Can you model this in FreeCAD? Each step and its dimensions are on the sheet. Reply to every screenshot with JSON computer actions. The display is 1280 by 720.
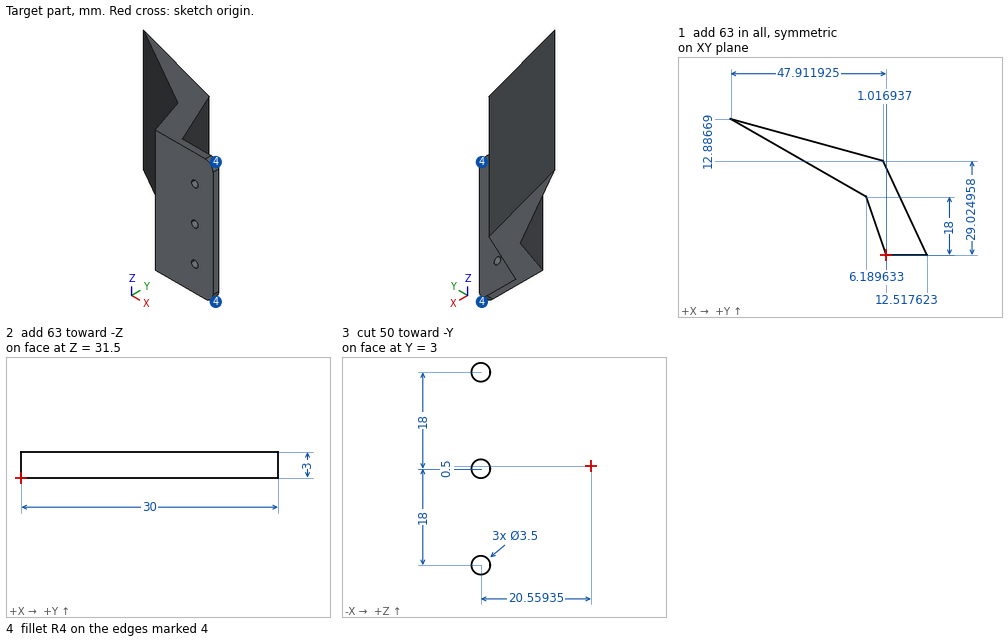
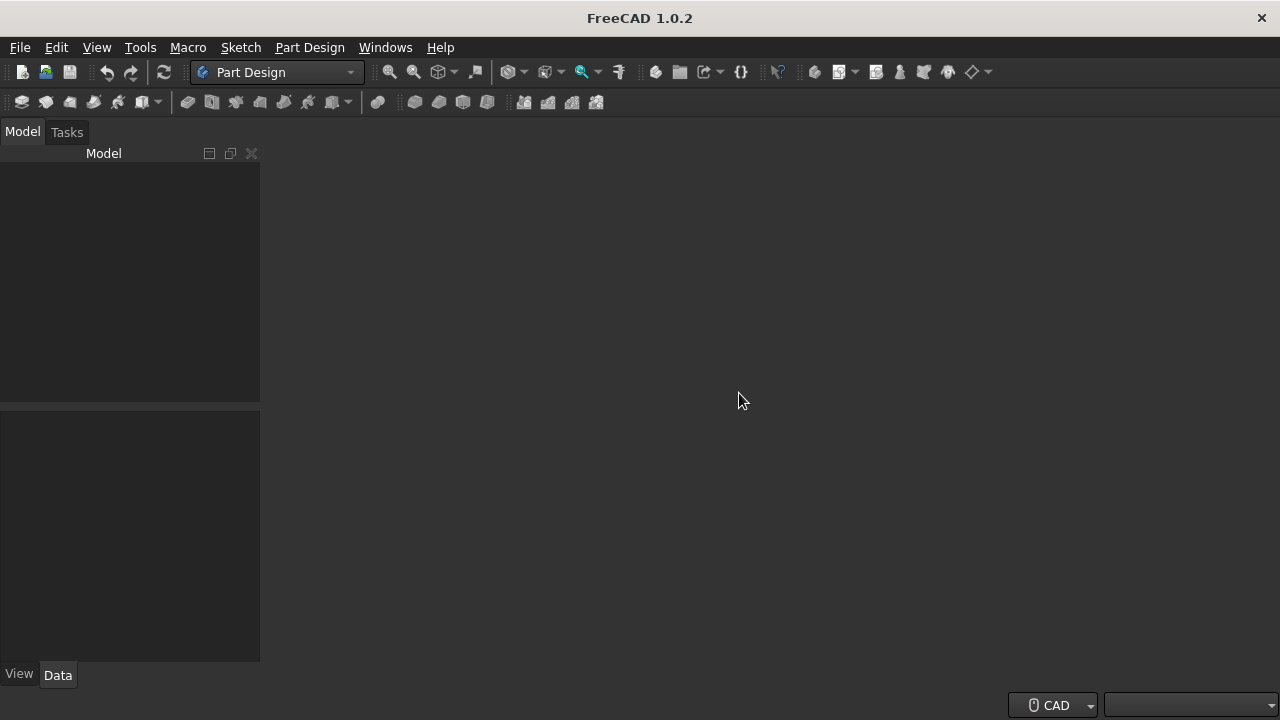
{"action": "key", "text": "ctrl+n"}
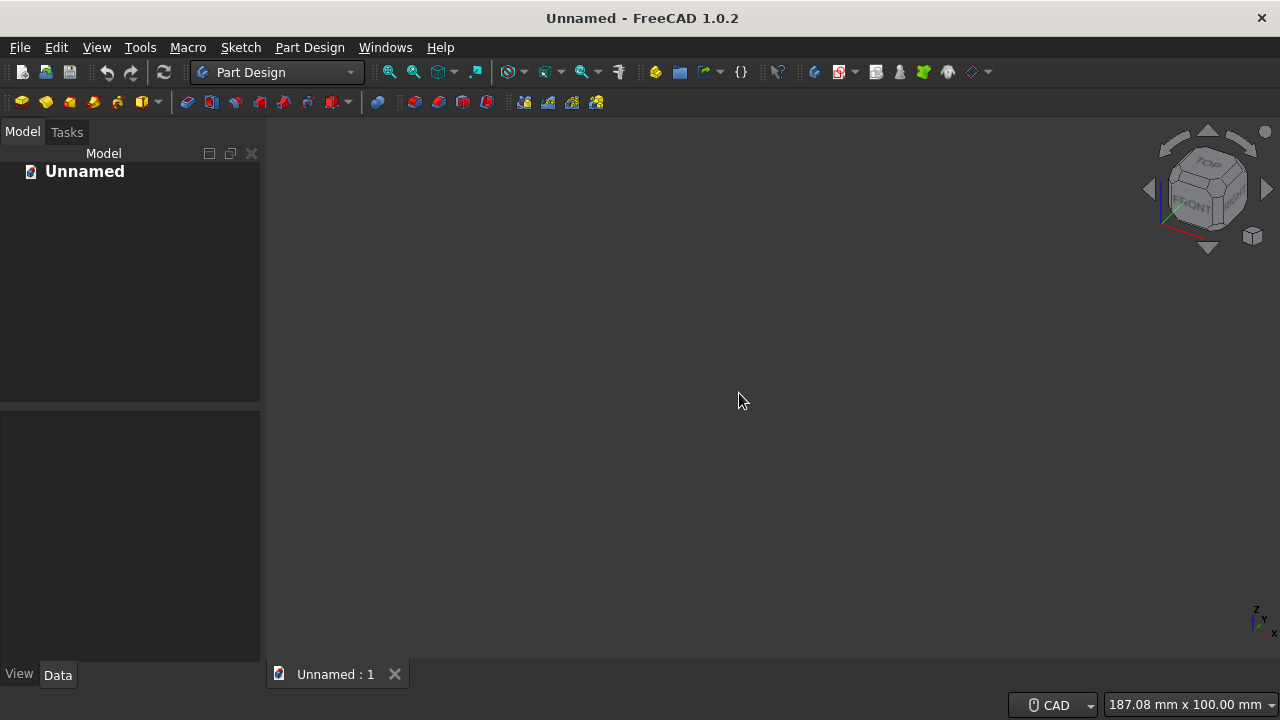
{"action": "left_click", "coordinate": [840, 72]}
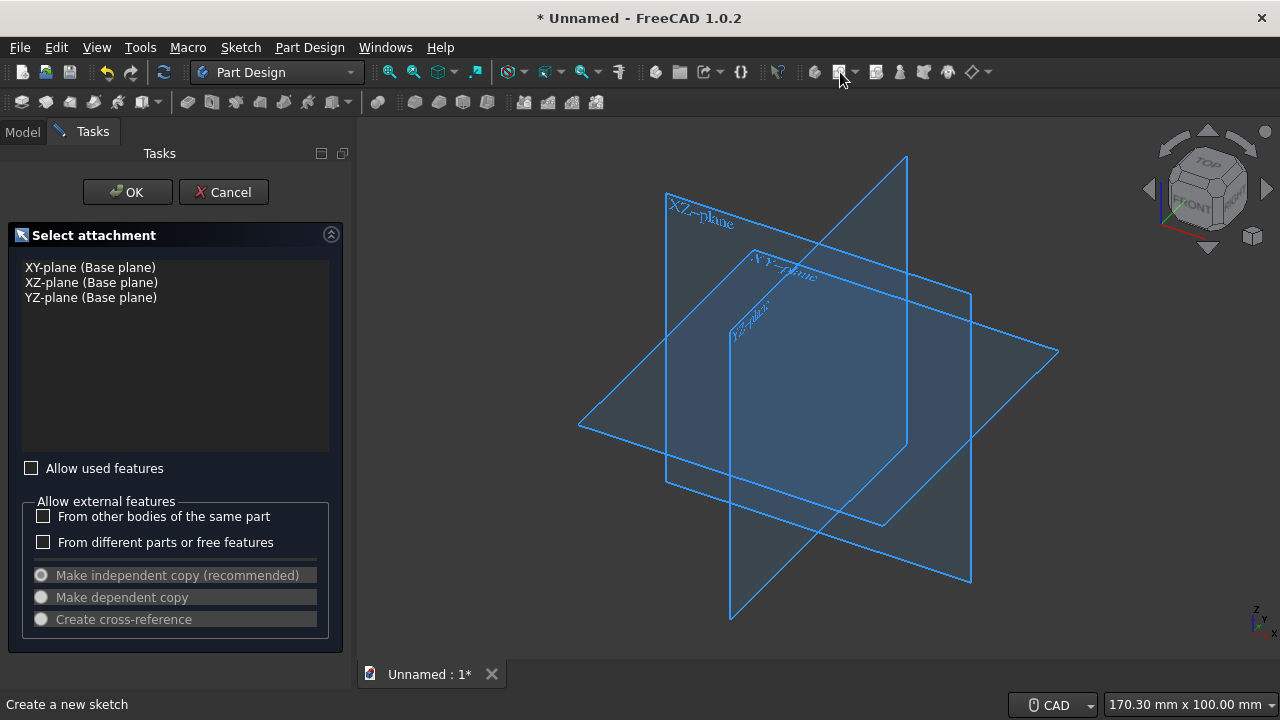
{"action": "left_click", "coordinate": [82, 268]}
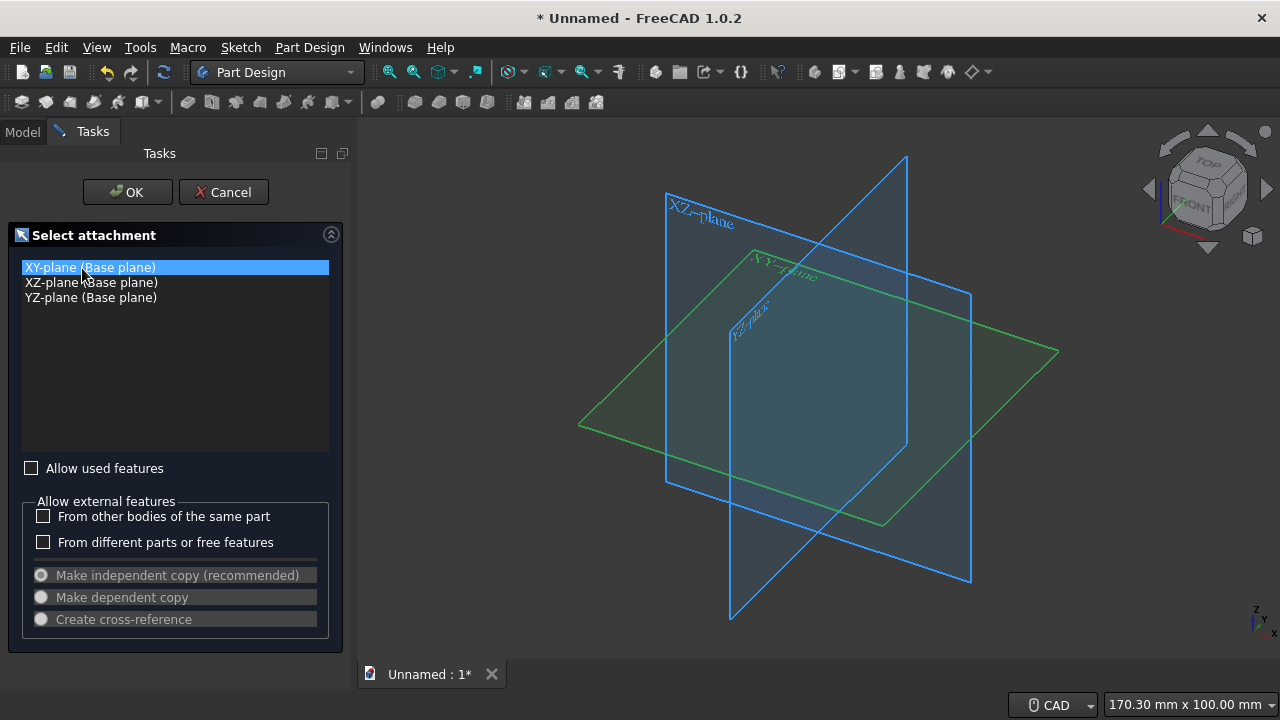
{"action": "left_click", "coordinate": [128, 192]}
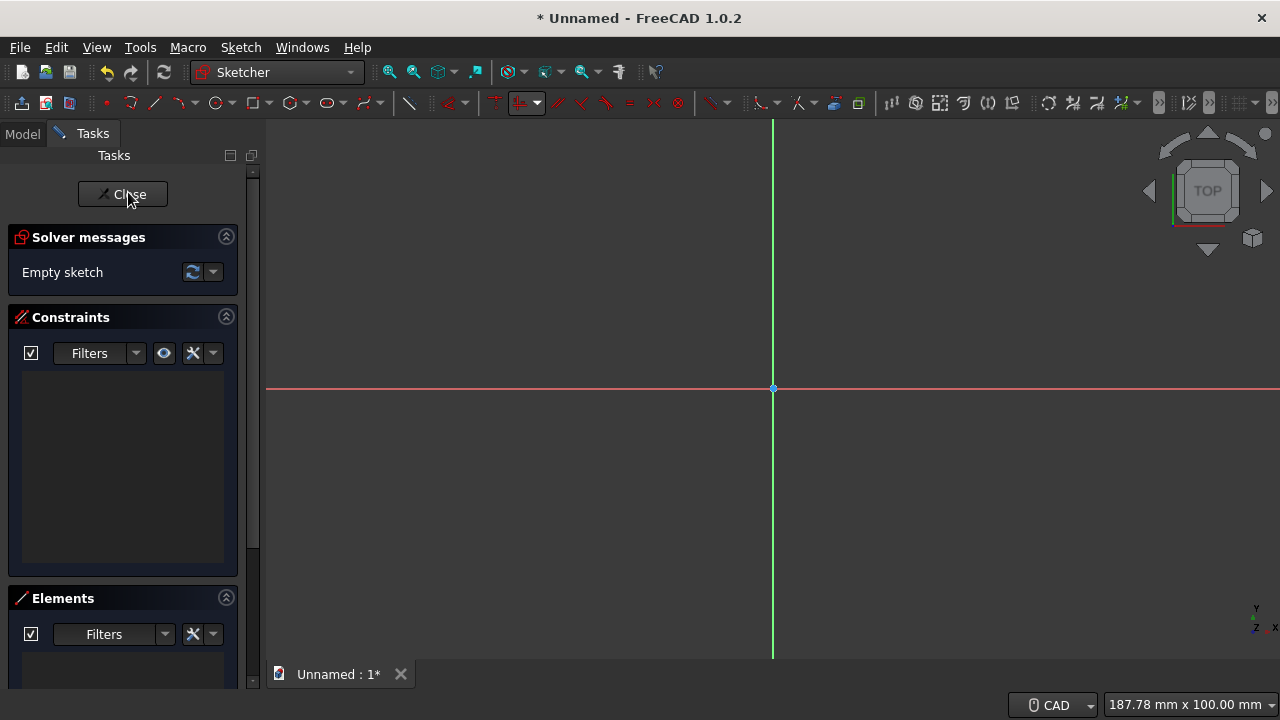
{"action": "scroll", "coordinate": [827, 631], "scroll_direction": "down", "scroll_amount": 1}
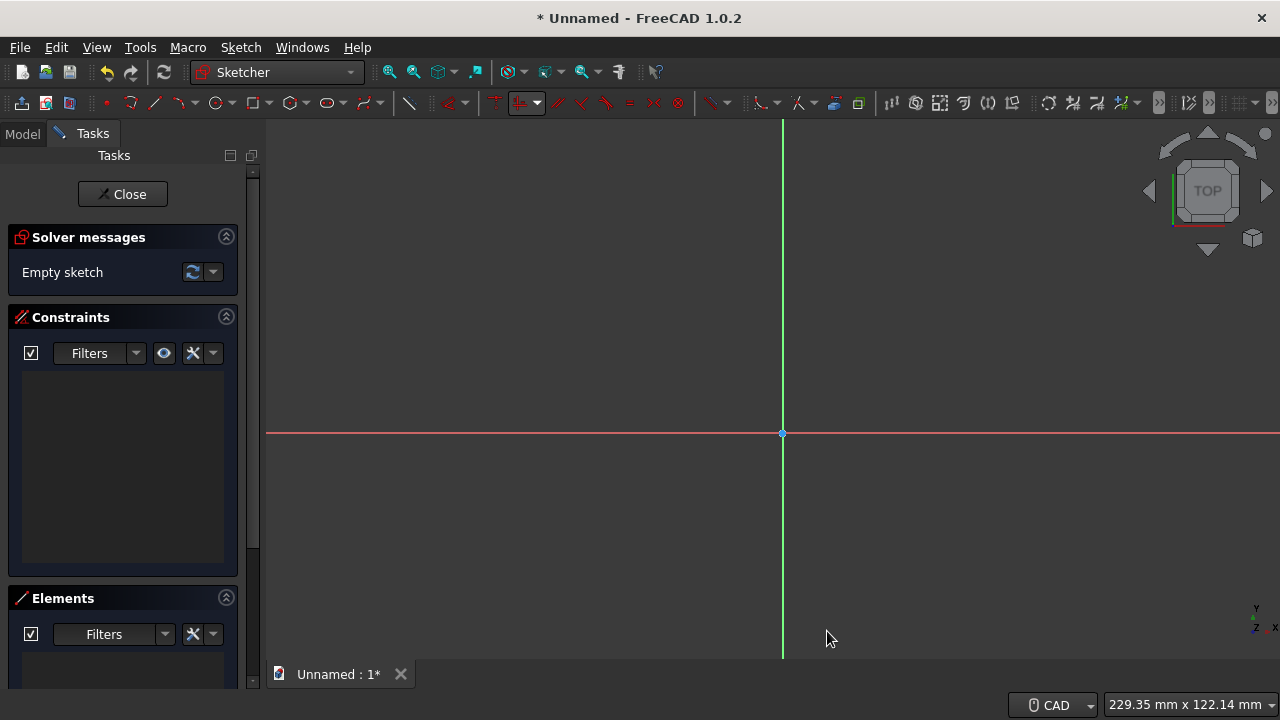
{"action": "scroll", "coordinate": [705, 281], "scroll_direction": "up", "scroll_amount": 3}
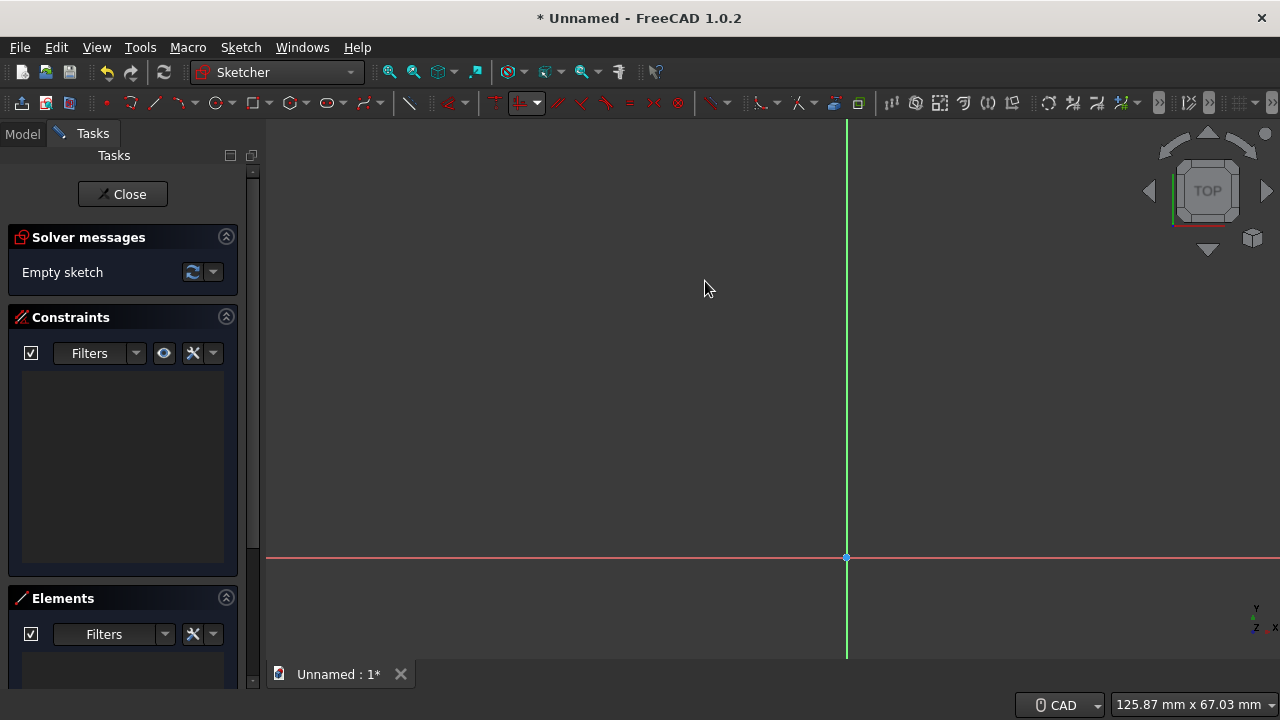
{"action": "key", "text": "g m"}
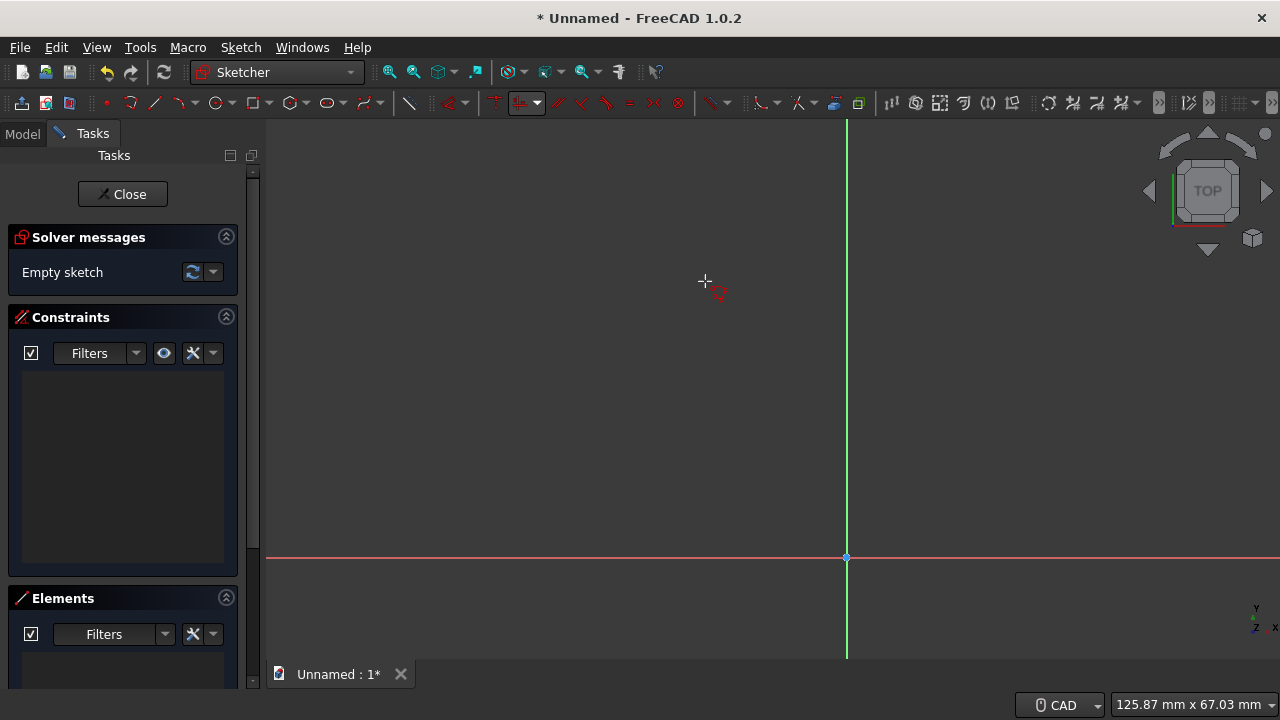
{"action": "left_click", "coordinate": [847, 558]}
{"action": "left_click", "coordinate": [947, 549]}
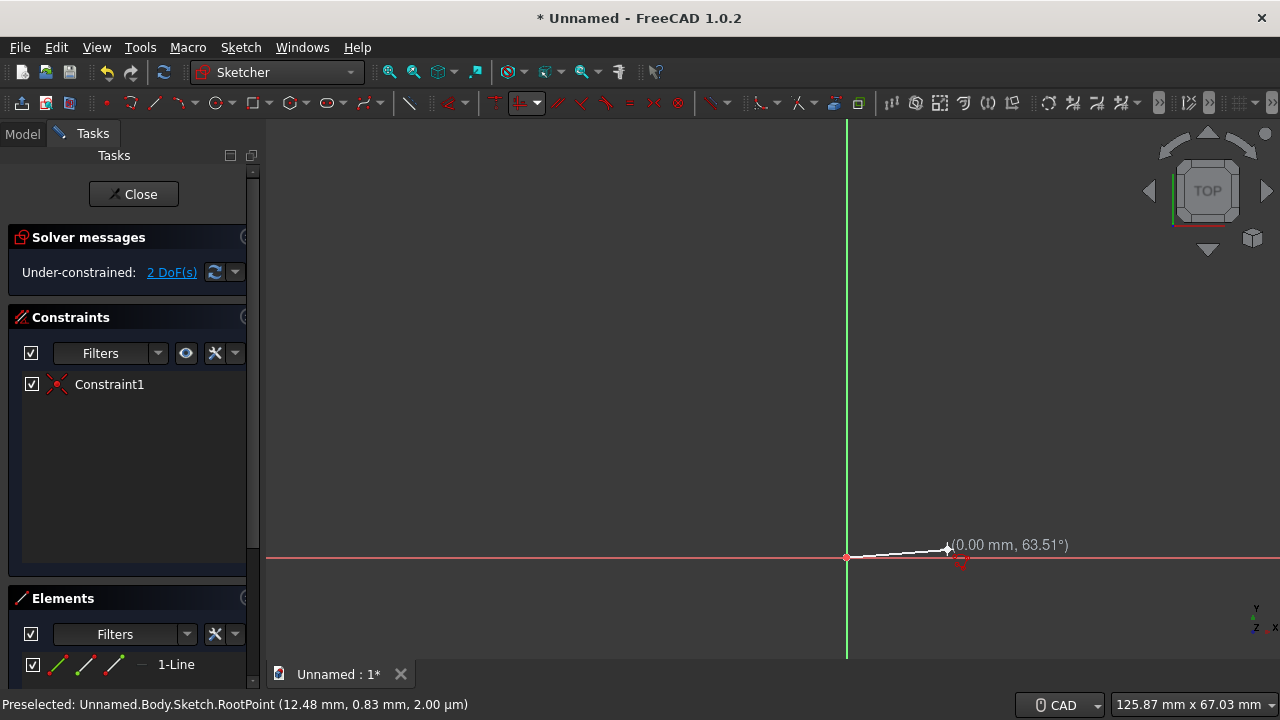
{"action": "scroll", "coordinate": [838, 324], "scroll_direction": "up", "scroll_amount": 4}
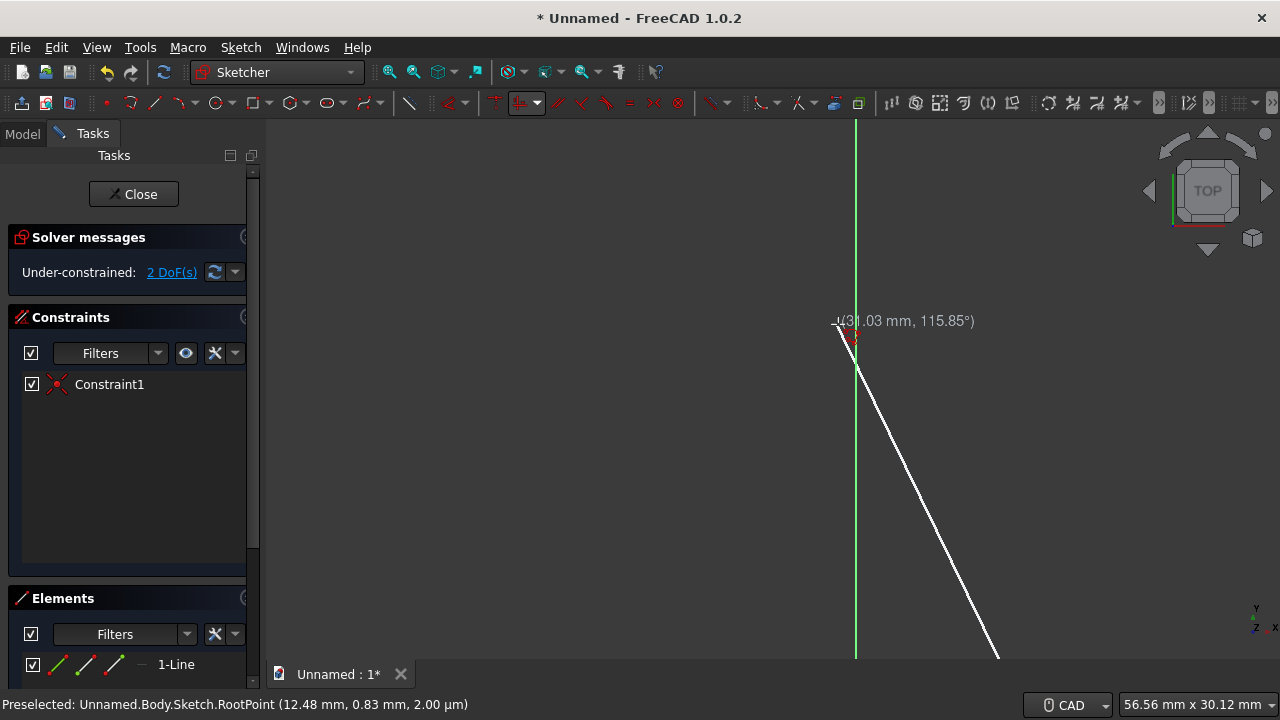
{"action": "left_click", "coordinate": [838, 323]}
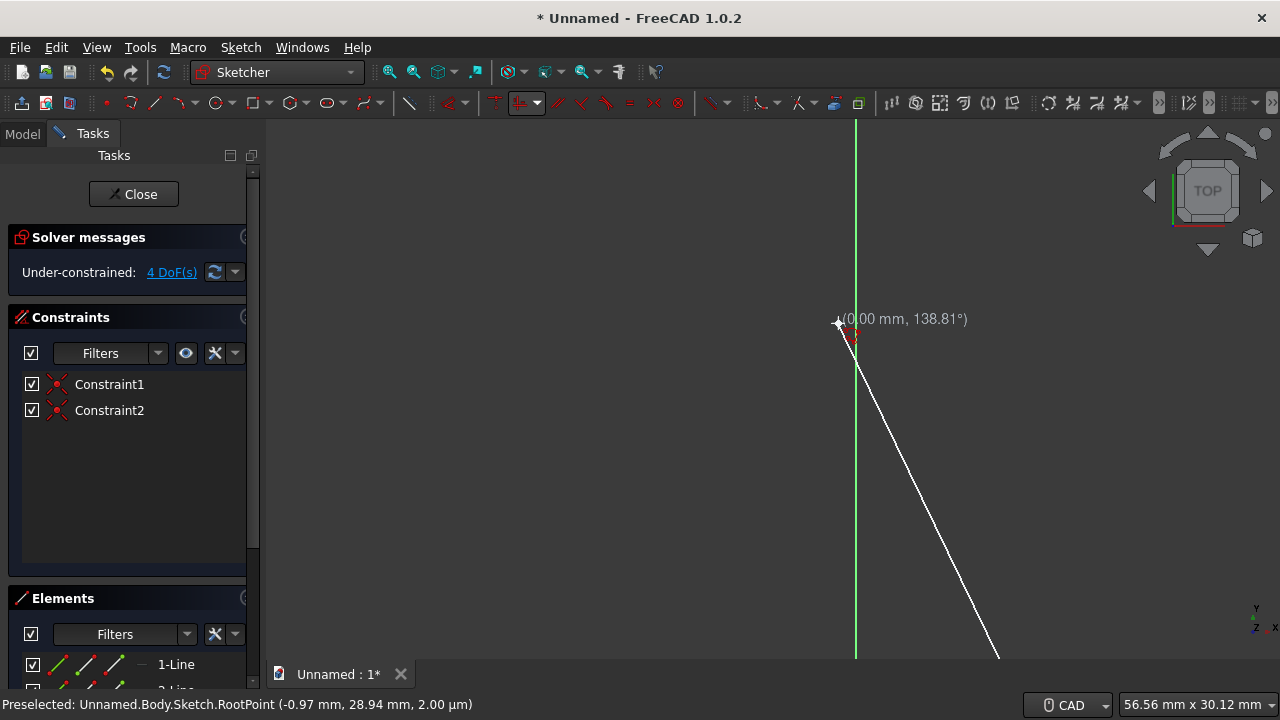
{"action": "scroll", "coordinate": [839, 324], "scroll_direction": "down", "scroll_amount": 4}